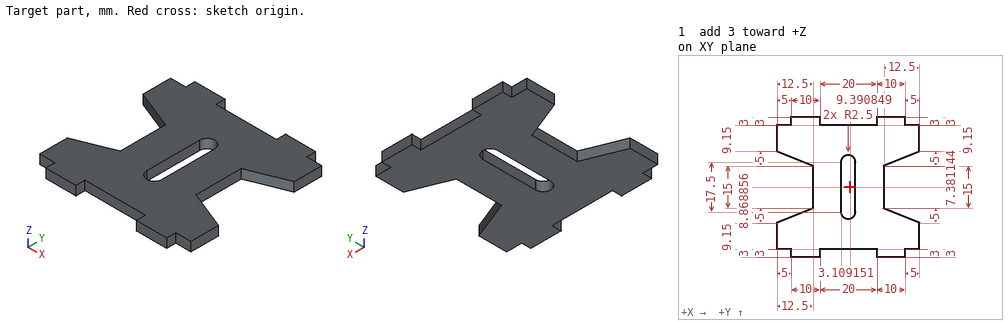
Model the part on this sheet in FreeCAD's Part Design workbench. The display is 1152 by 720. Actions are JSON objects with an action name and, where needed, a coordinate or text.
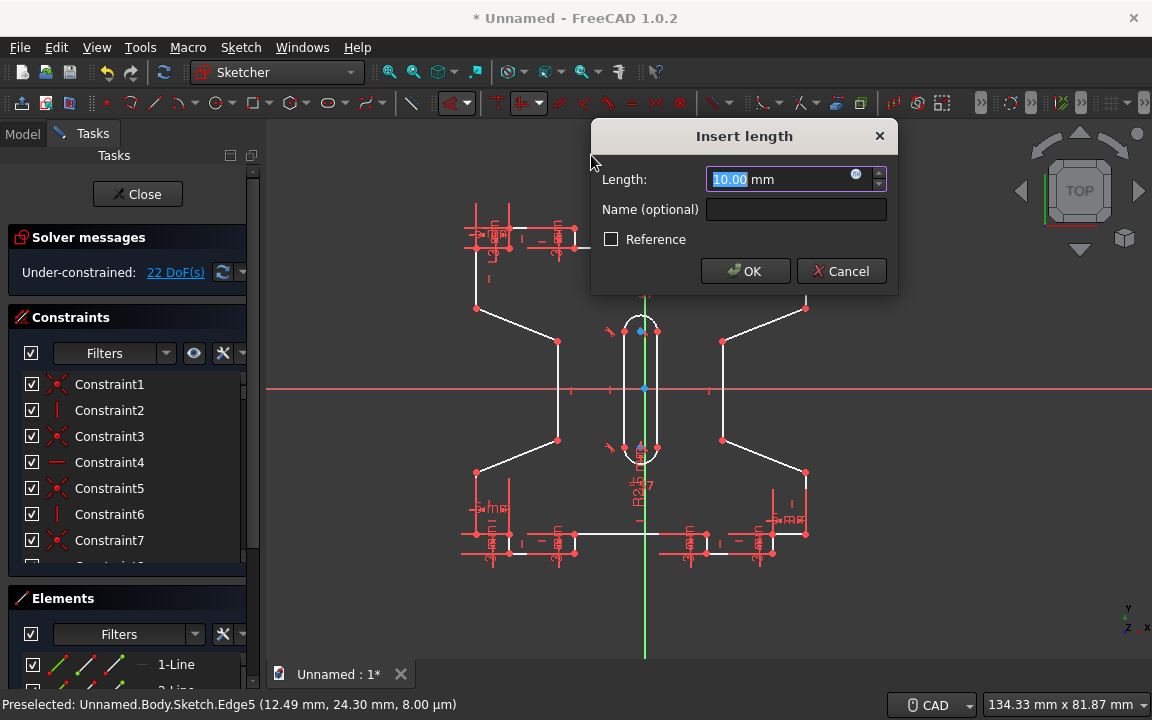
{"action": "type", "text": "10"}
{"action": "key", "text": "Return"}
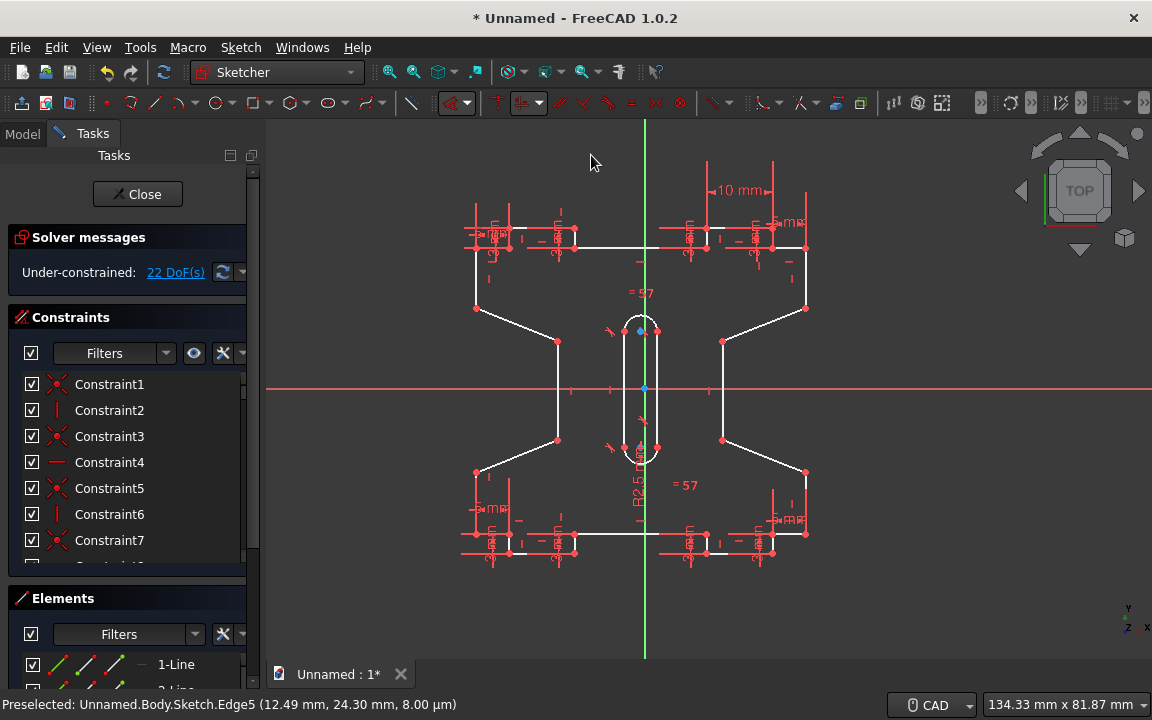
{"action": "left_click", "coordinate": [667, 248]}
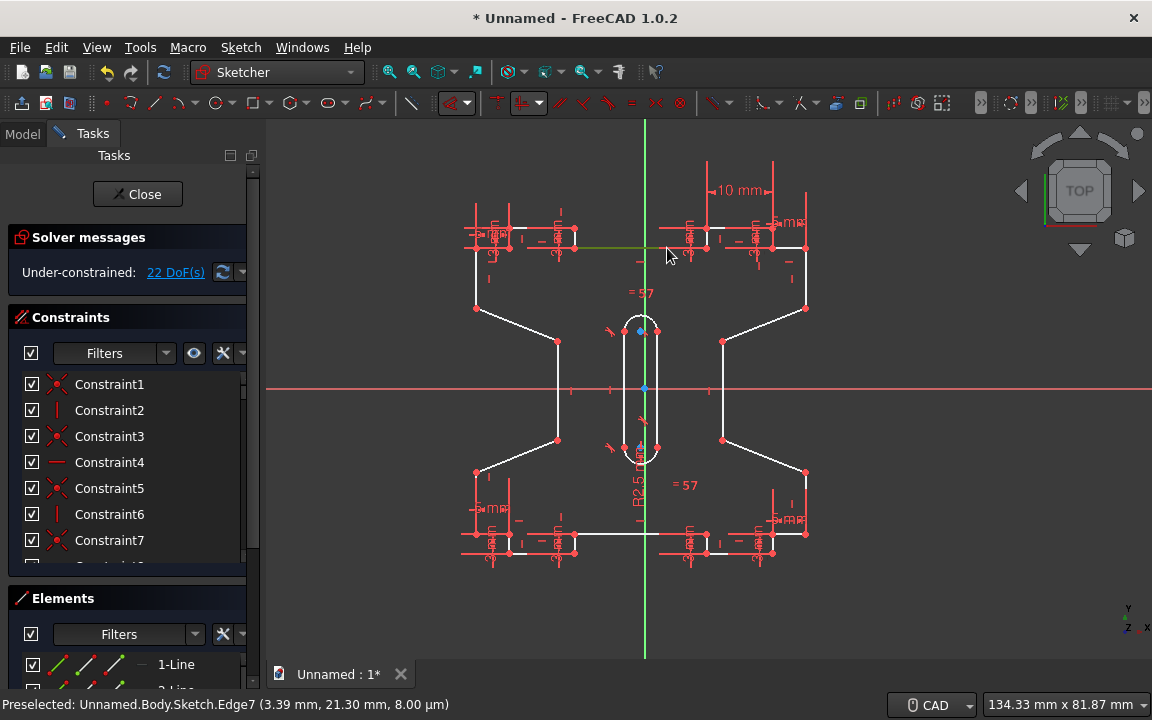
{"action": "key", "text": "l"}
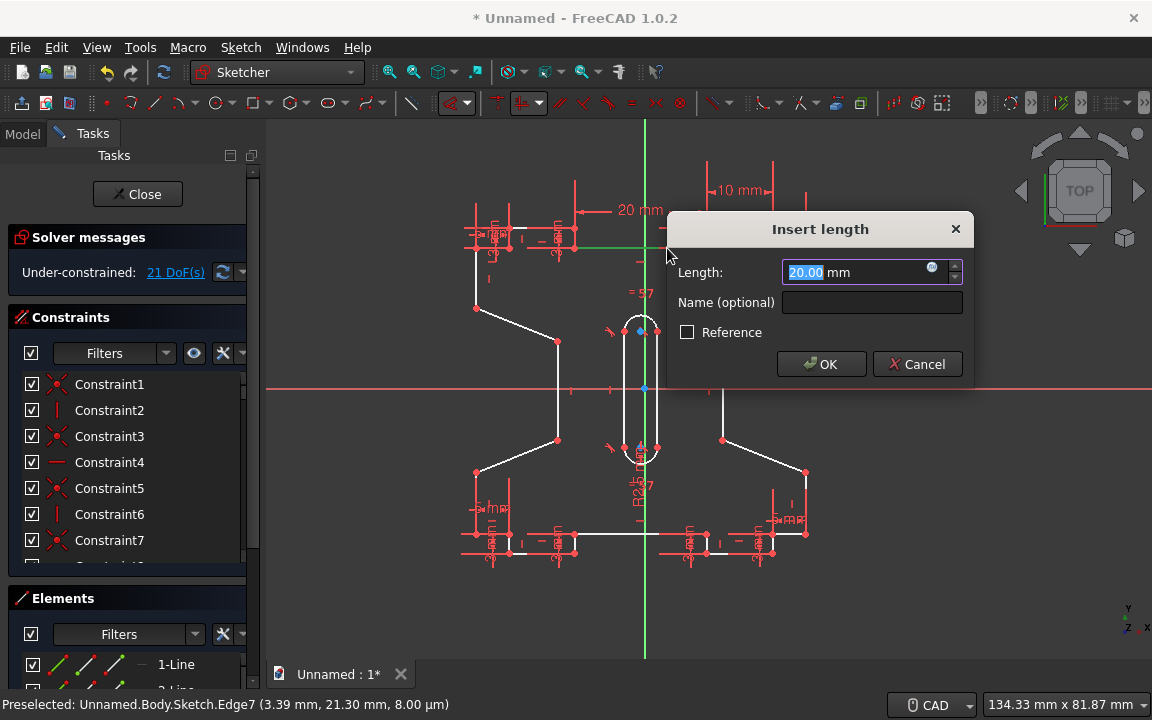
{"action": "type", "text": "20"}
{"action": "key", "text": "Return"}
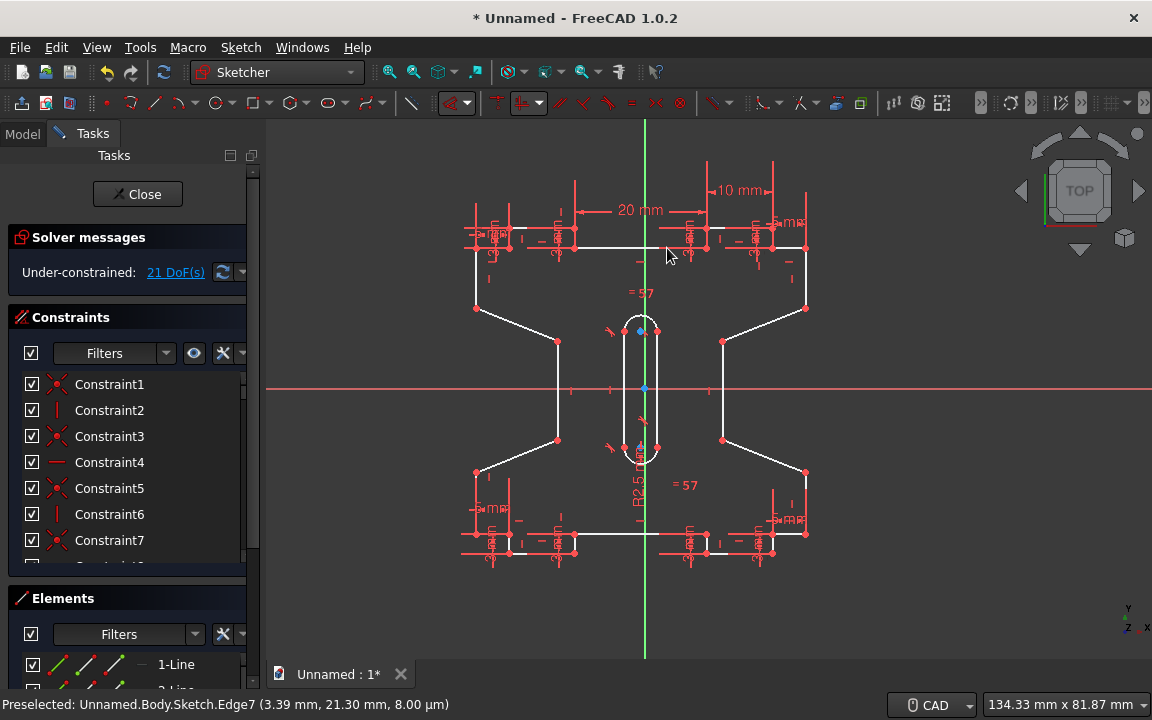
{"action": "left_click", "coordinate": [529, 228]}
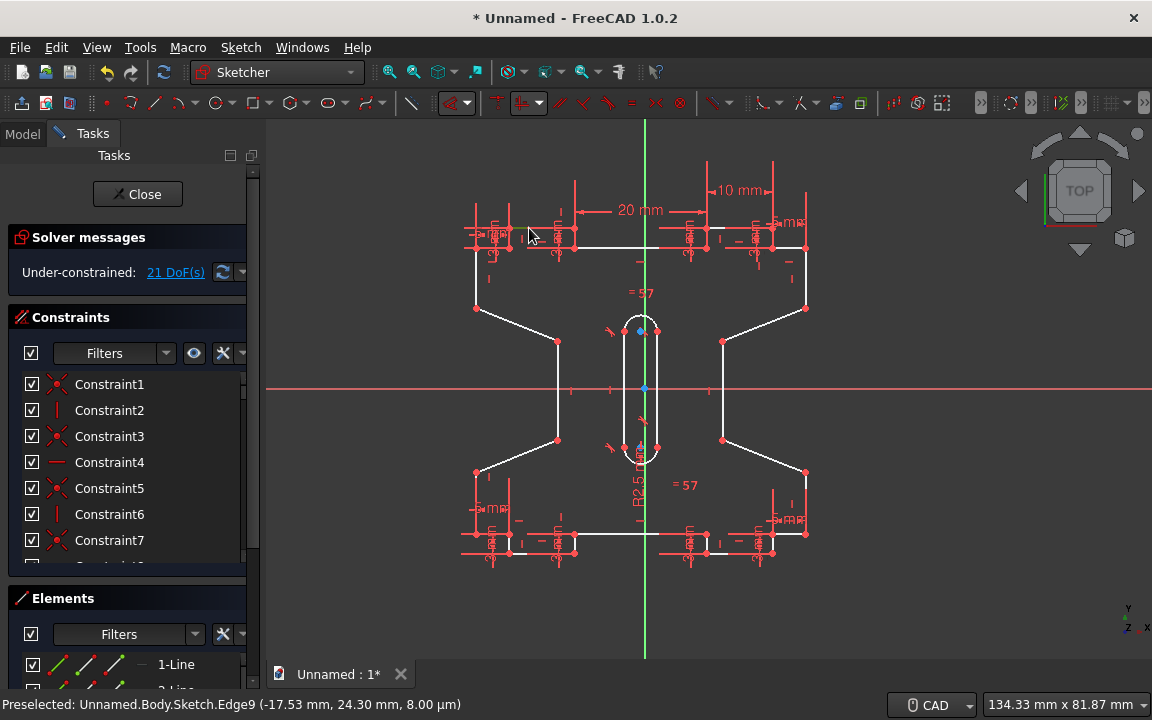
{"action": "key", "text": "l"}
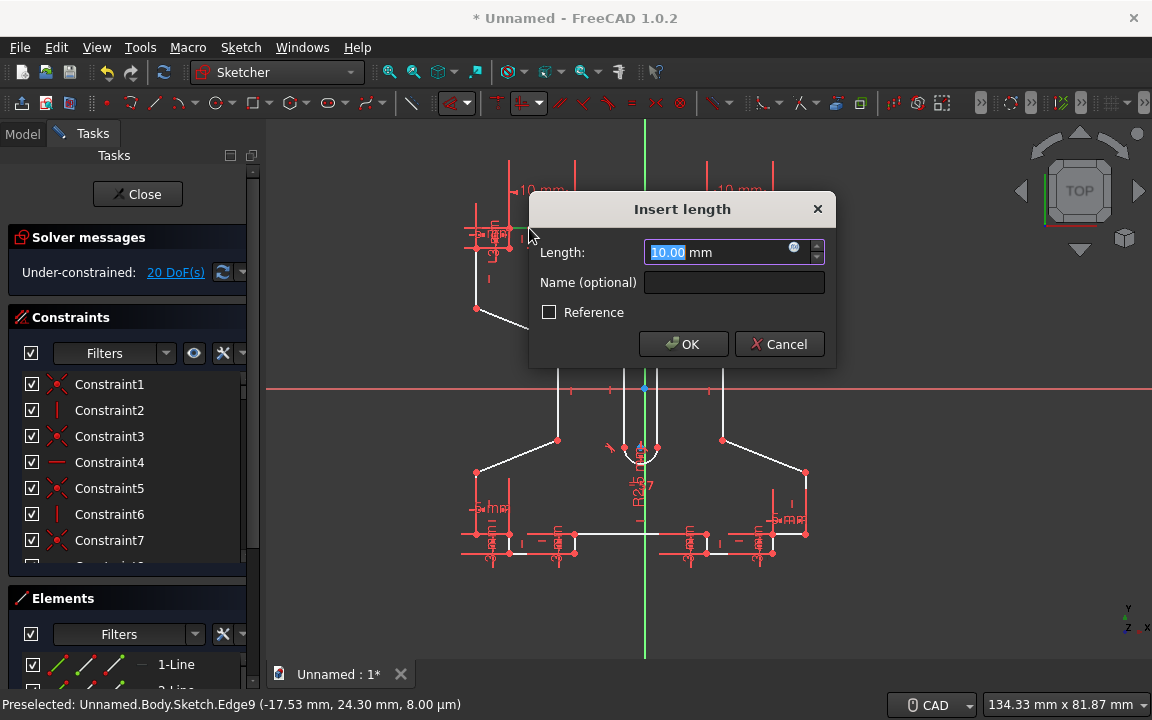
{"action": "type", "text": "10"}
{"action": "key", "text": "Return"}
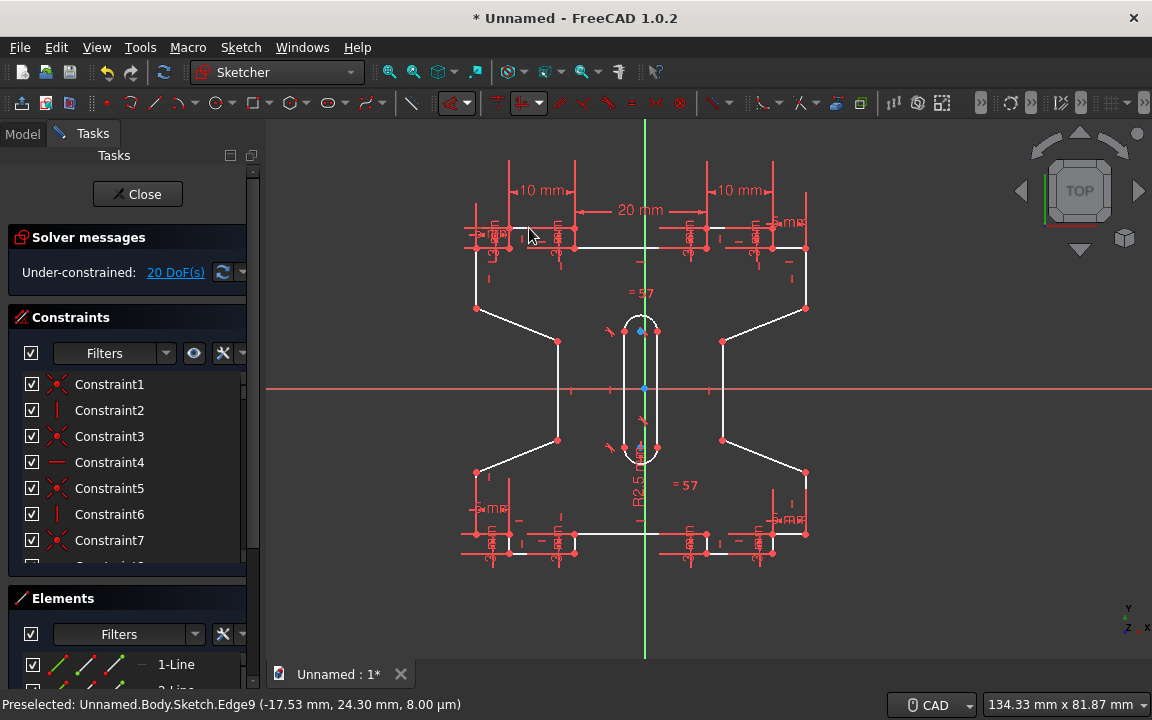
{"action": "left_click", "coordinate": [558, 371]}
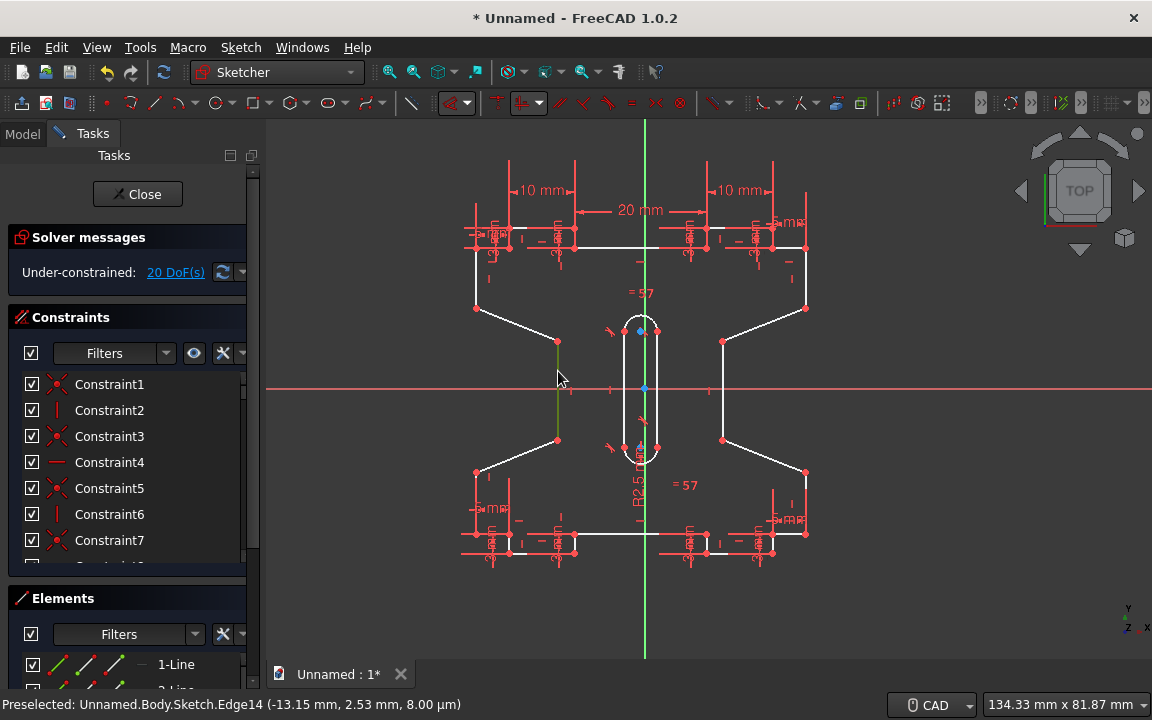
{"action": "key", "text": "i"}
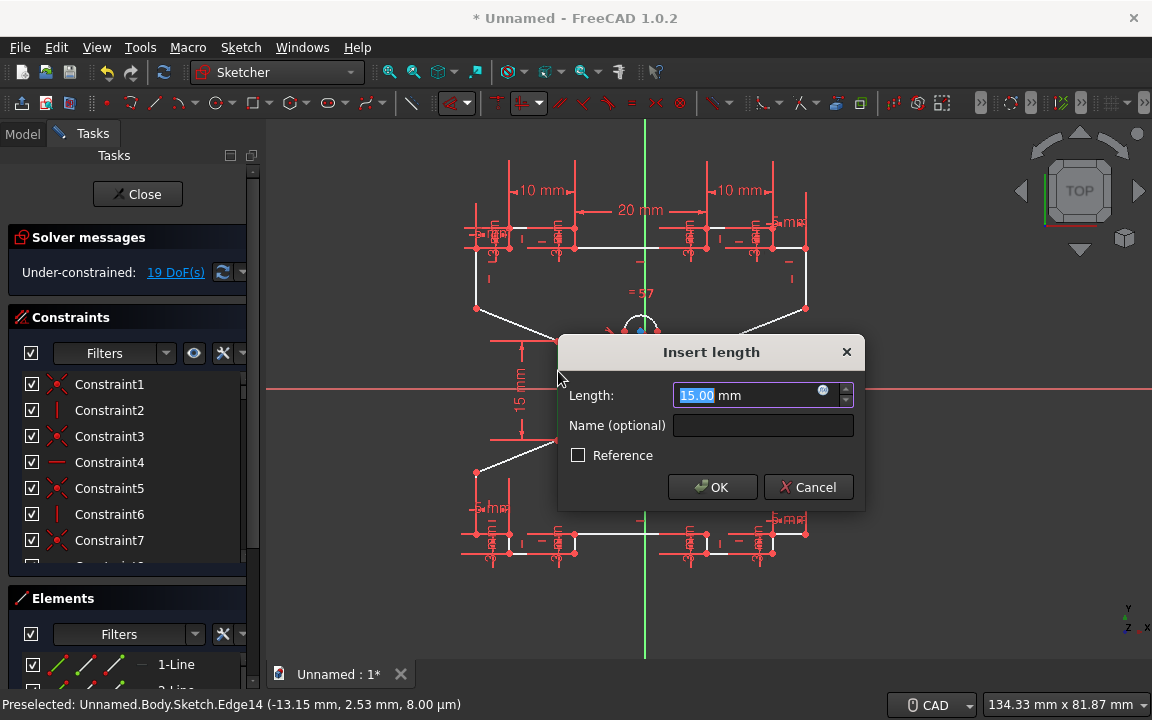
{"action": "type", "text": "15"}
{"action": "key", "text": "Return"}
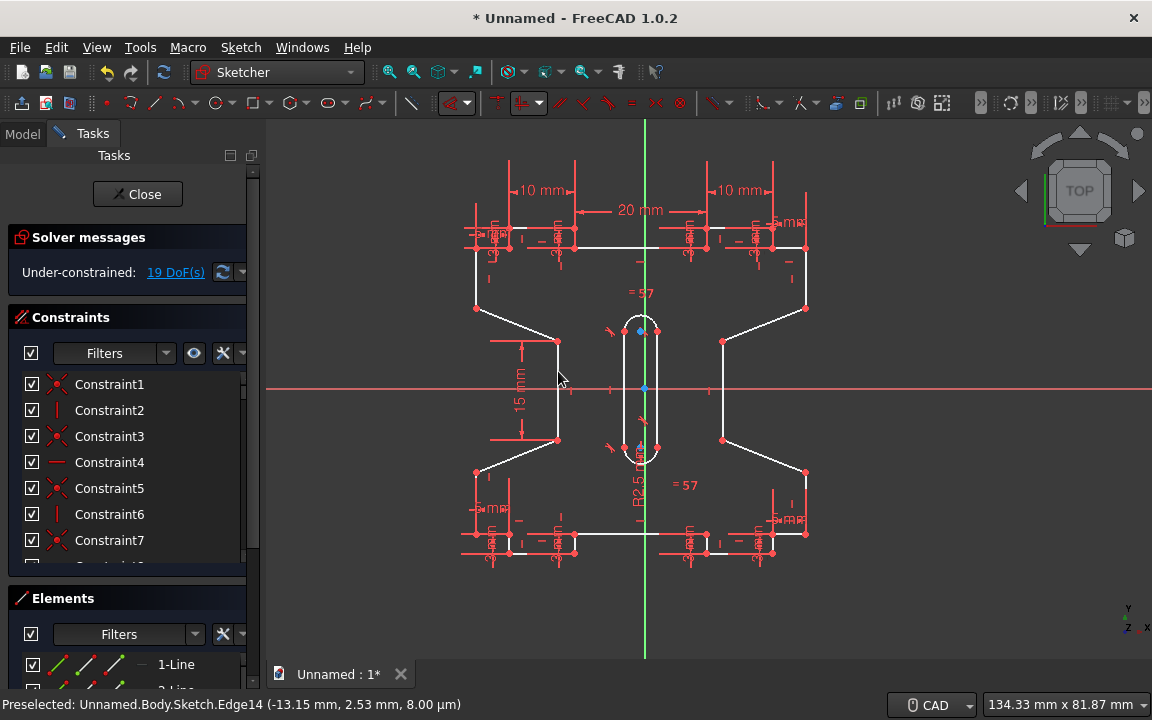
{"action": "left_click", "coordinate": [529, 554]}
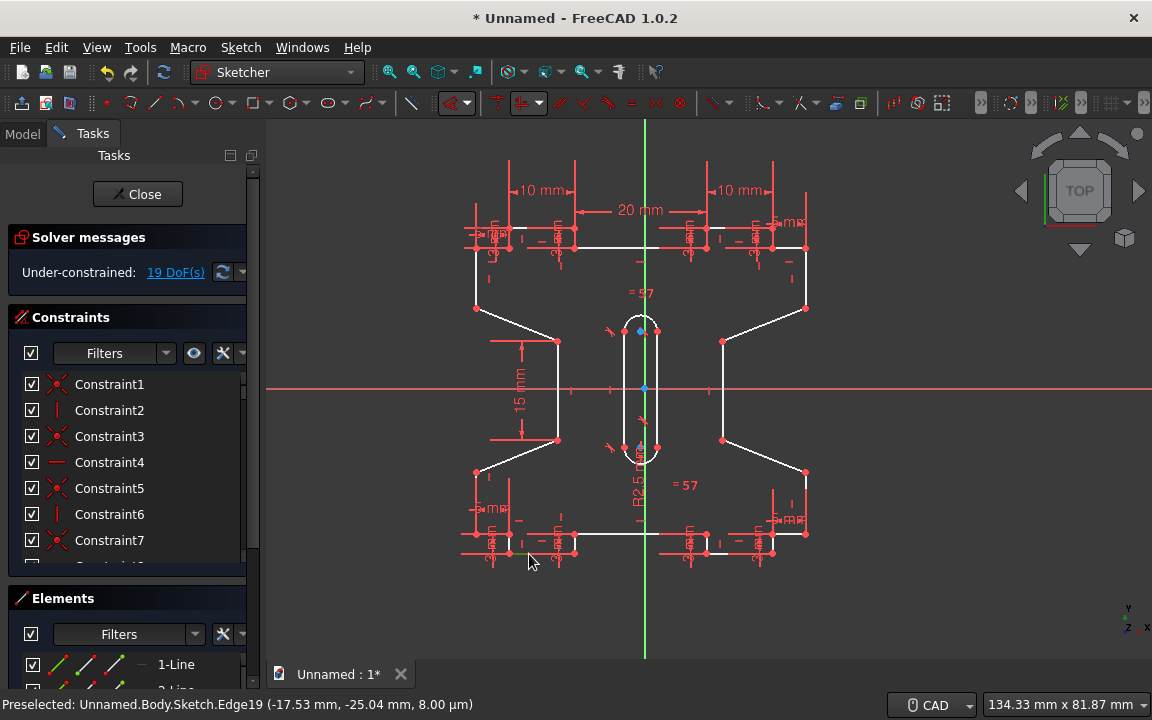
{"action": "left_click", "coordinate": [470, 104]}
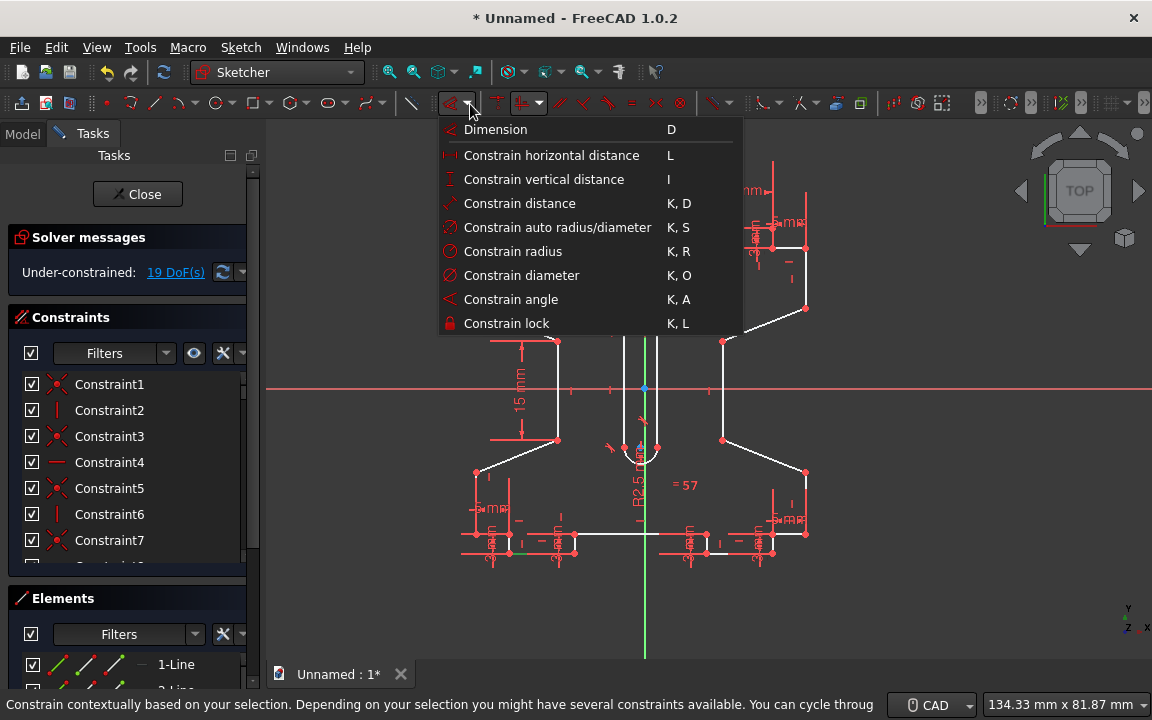
{"action": "left_click", "coordinate": [591, 155]}